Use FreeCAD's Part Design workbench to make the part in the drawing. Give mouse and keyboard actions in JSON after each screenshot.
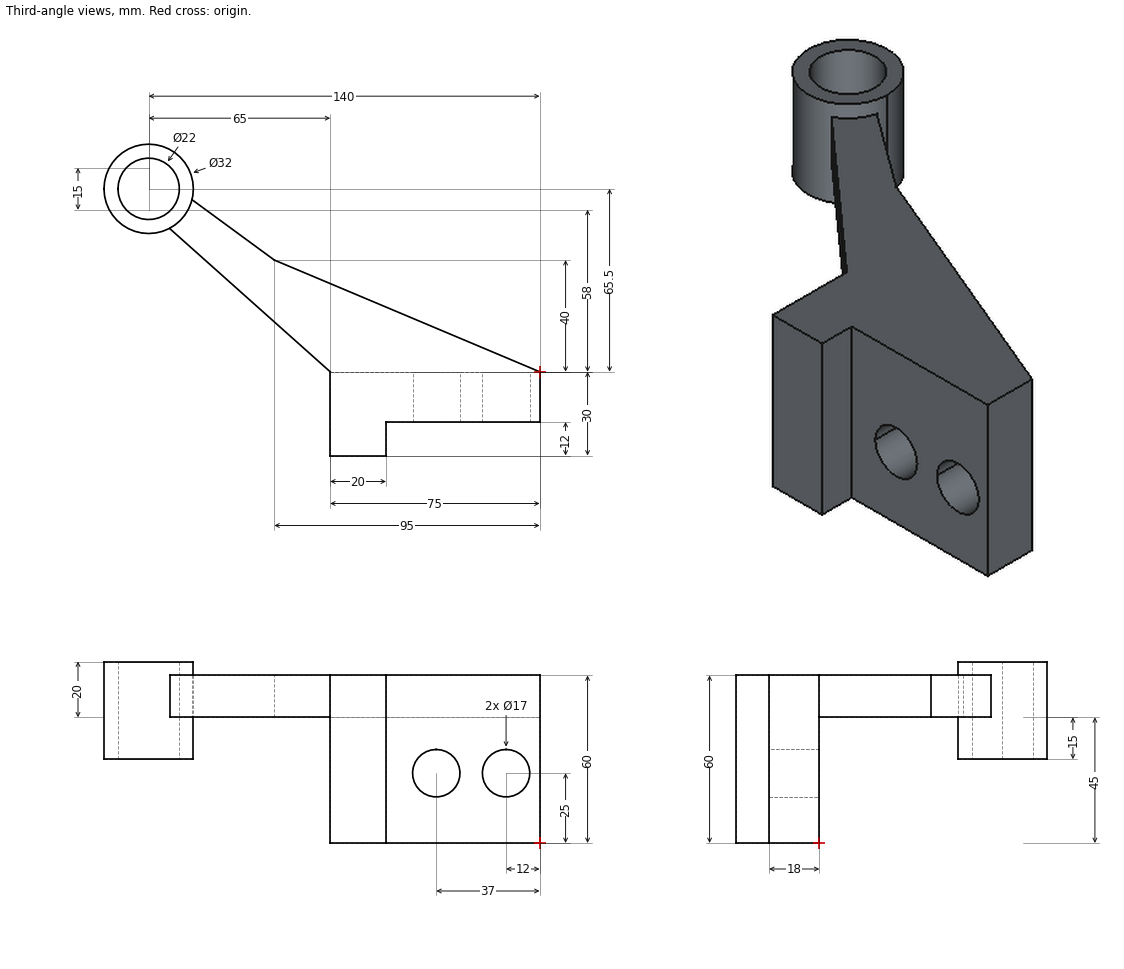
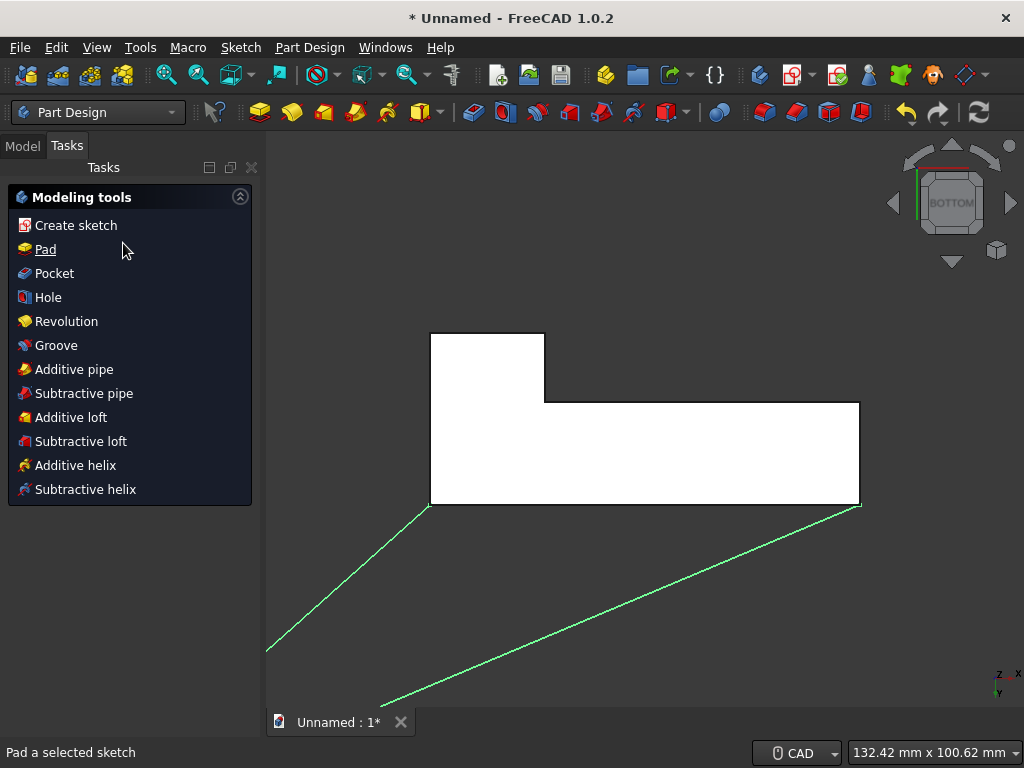
{"action": "left_click", "coordinate": [260, 112]}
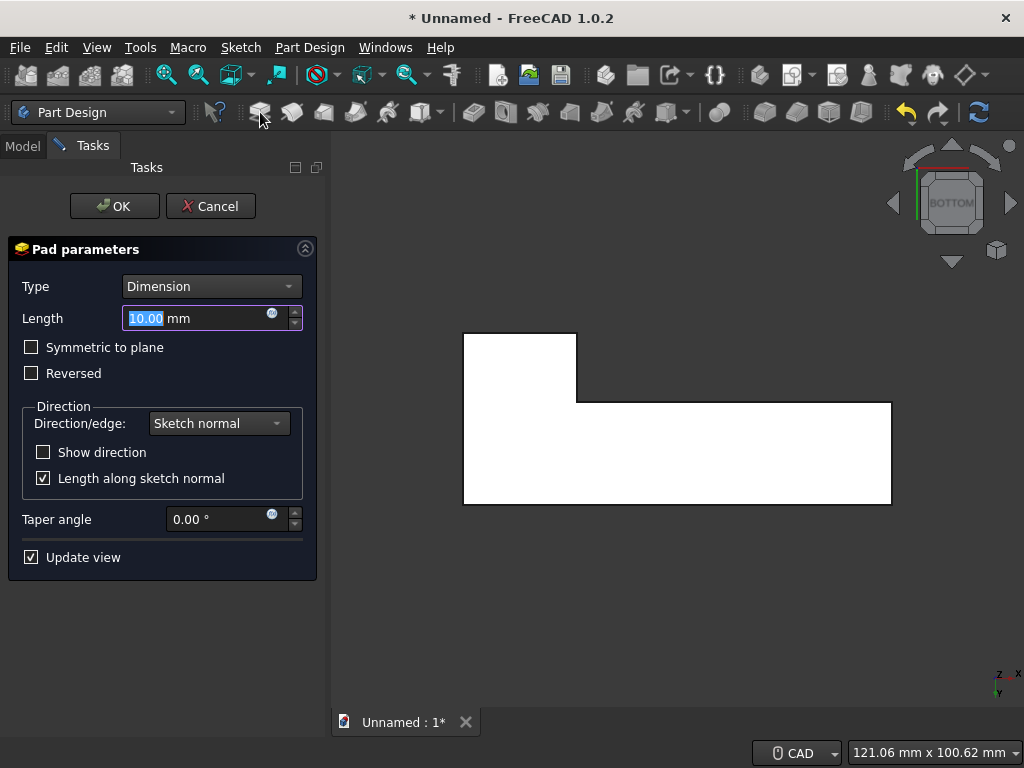
{"action": "type", "text": "60"}
{"action": "key", "text": "Tab"}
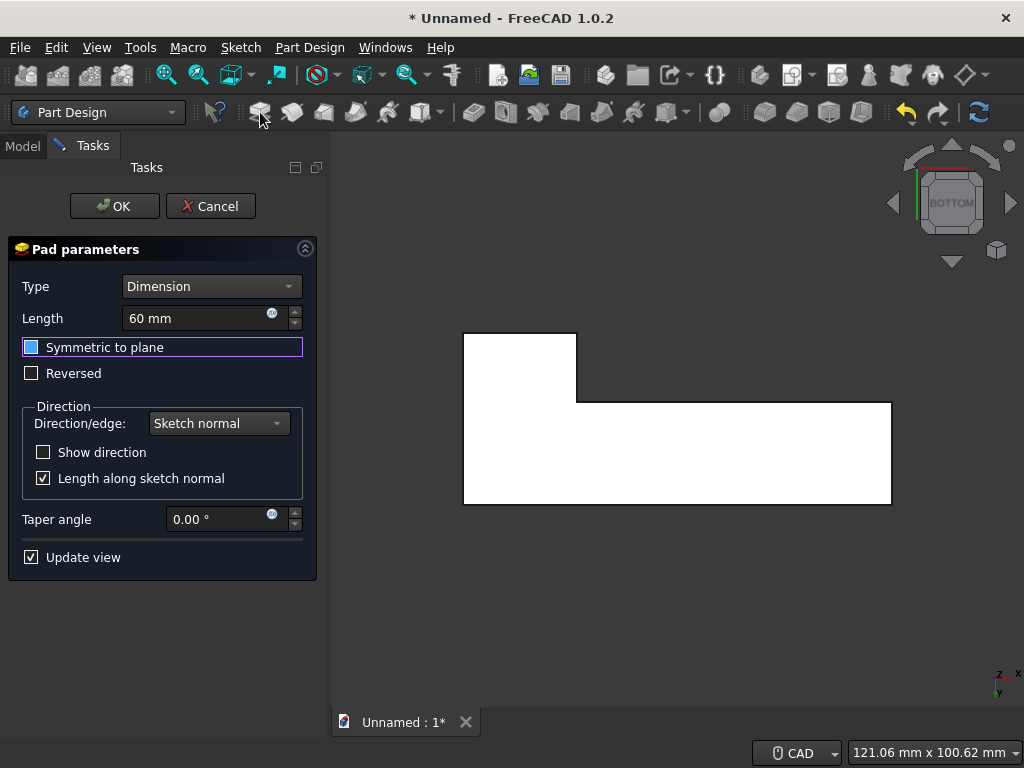
{"action": "left_click", "coordinate": [30, 373]}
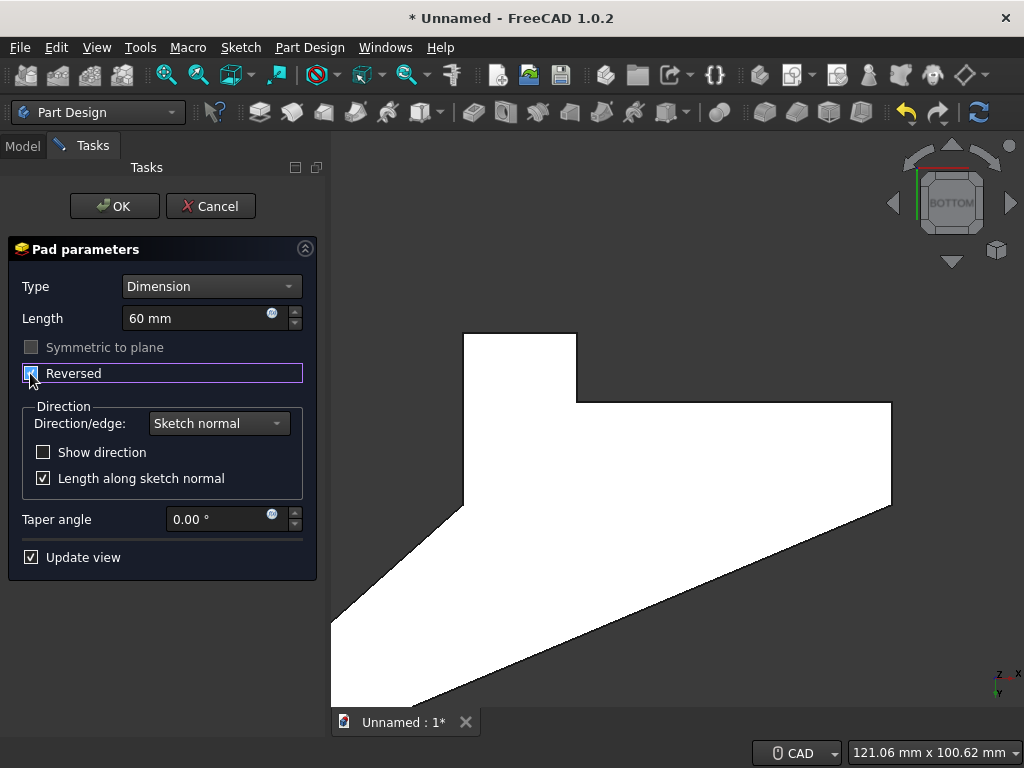
{"action": "left_click", "coordinate": [115, 206]}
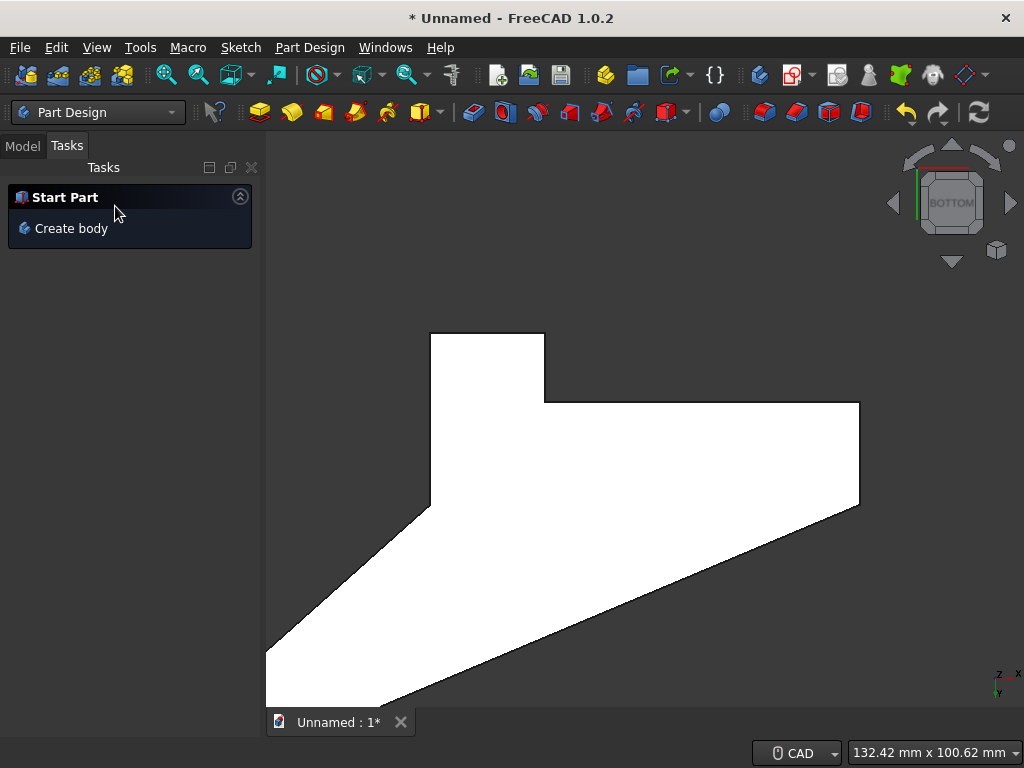
{"action": "left_click", "coordinate": [168, 76]}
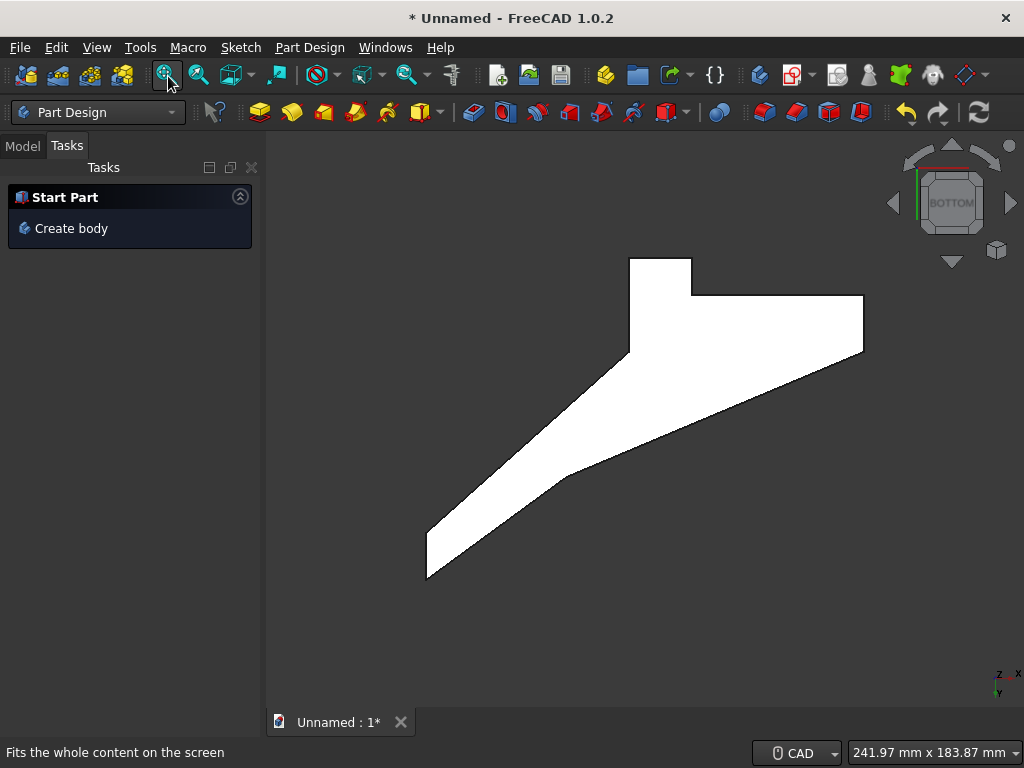
{"action": "left_click", "coordinate": [792, 76]}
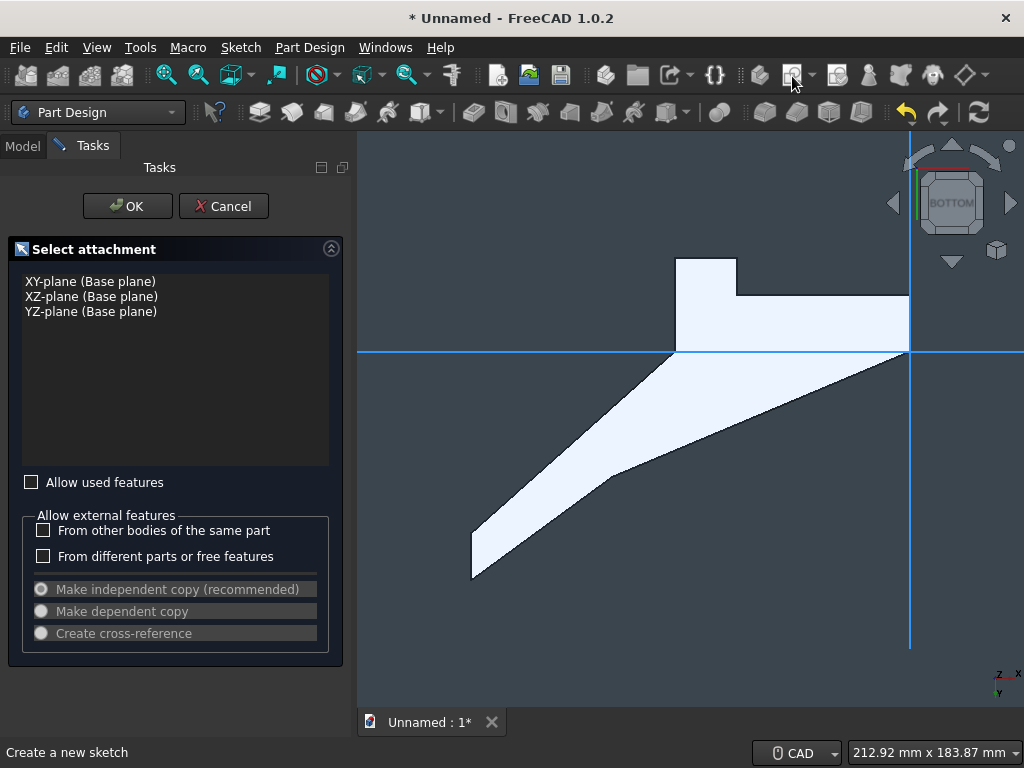
{"action": "left_click", "coordinate": [82, 282]}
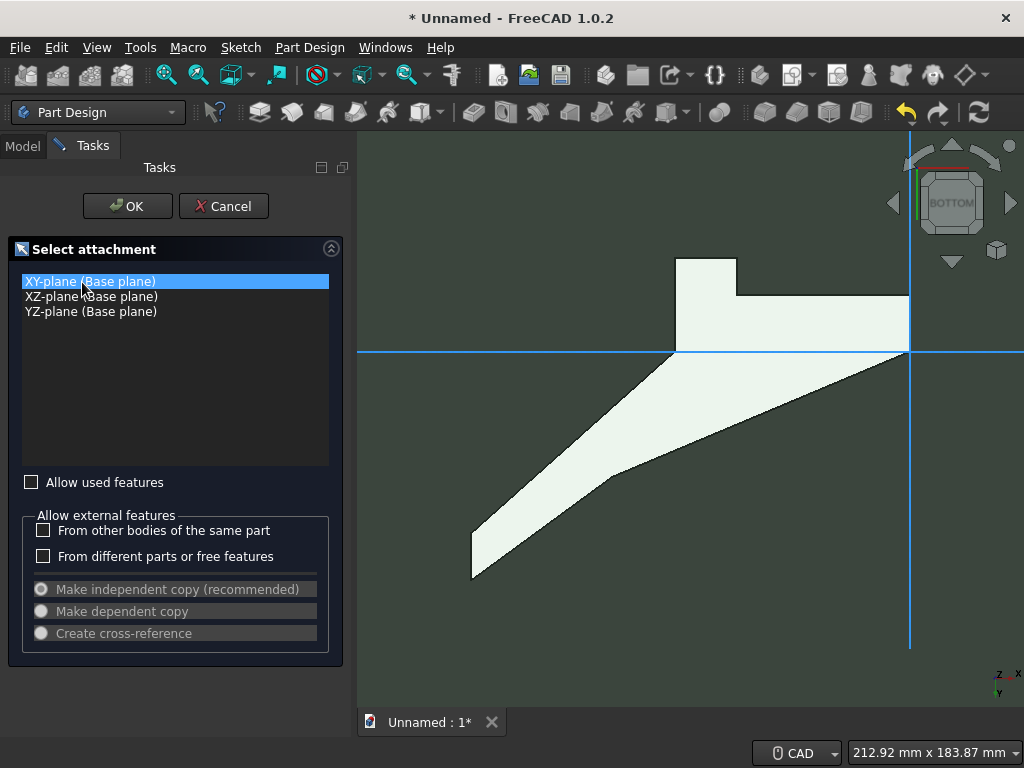
{"action": "left_click", "coordinate": [128, 206]}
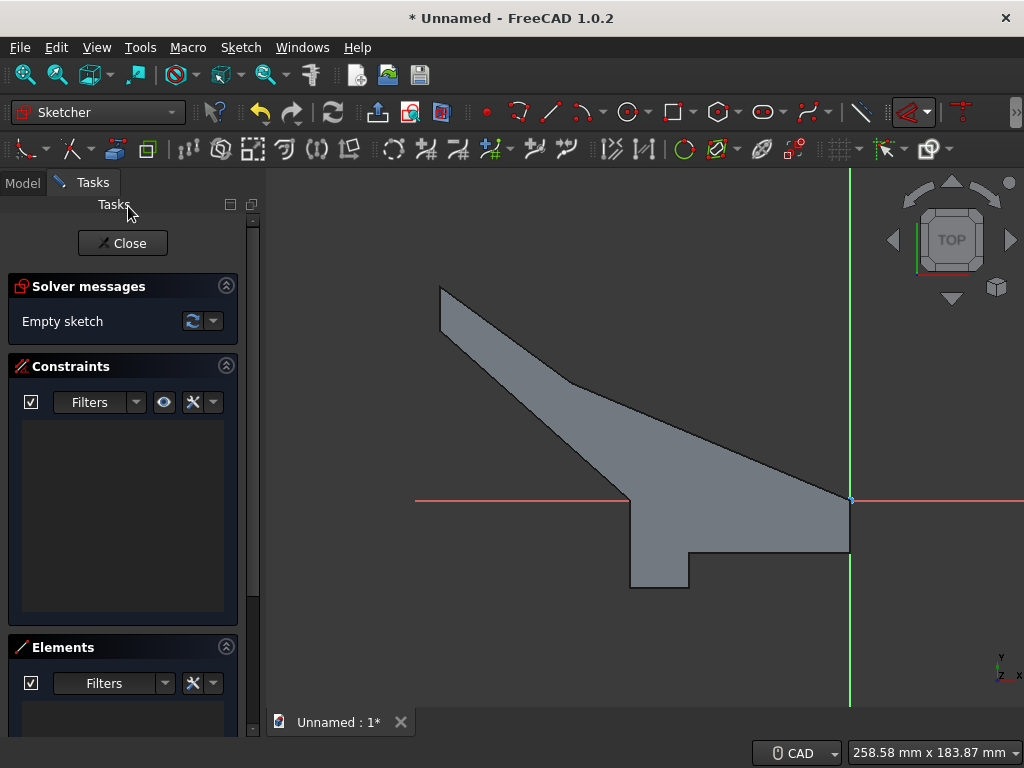
{"action": "left_click", "coordinate": [442, 112]}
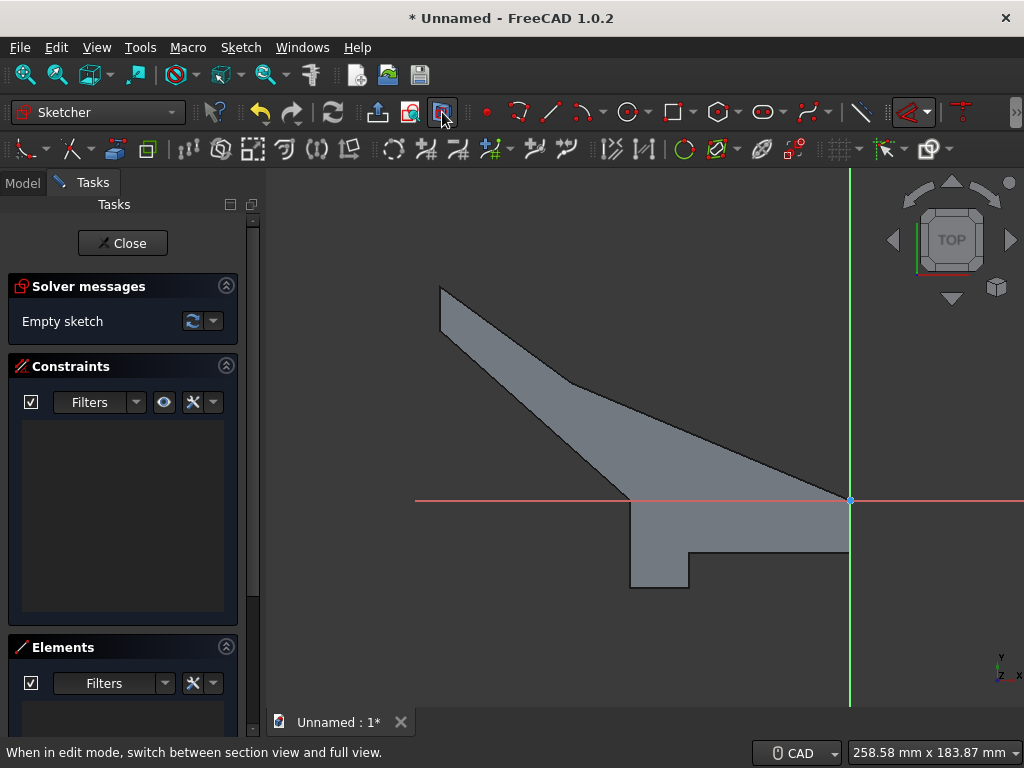
{"action": "scroll", "coordinate": [294, 636], "scroll_direction": "down", "scroll_amount": 1}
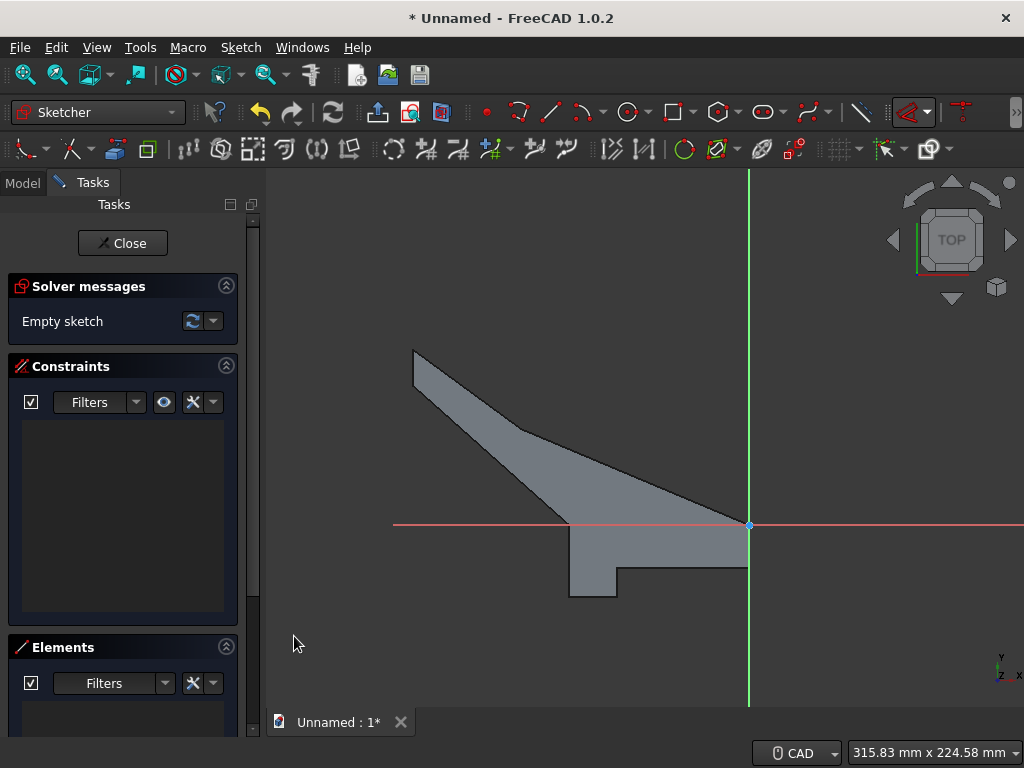
{"action": "left_click", "coordinate": [520, 112]}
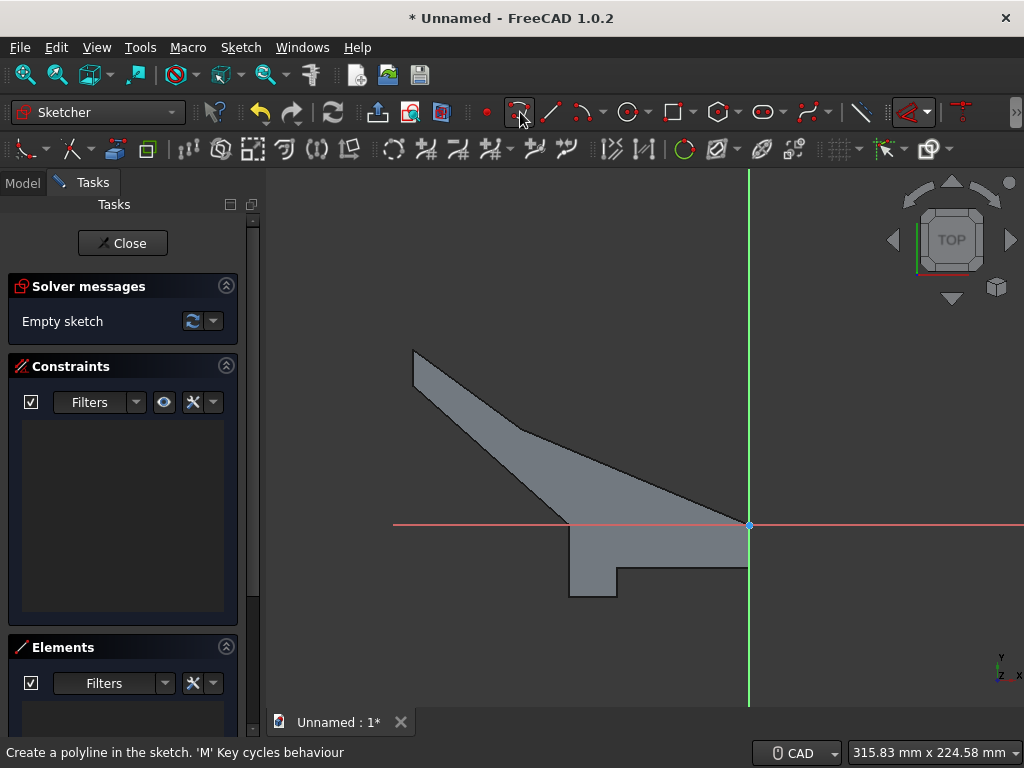
{"action": "left_click", "coordinate": [749, 525]}
{"action": "left_click", "coordinate": [569, 516]}
{"action": "left_click", "coordinate": [413, 386]}
{"action": "left_click", "coordinate": [413, 350]}
{"action": "left_click", "coordinate": [521, 429]}
{"action": "left_click", "coordinate": [749, 525]}
{"action": "key", "text": "Escape"}
{"action": "key", "text": "Escape"}